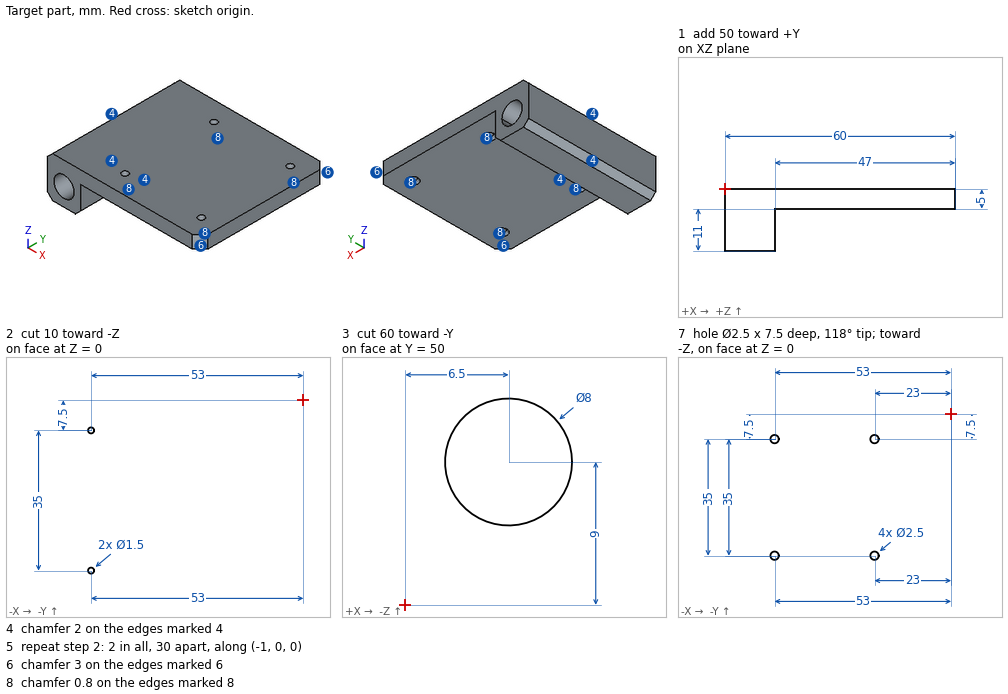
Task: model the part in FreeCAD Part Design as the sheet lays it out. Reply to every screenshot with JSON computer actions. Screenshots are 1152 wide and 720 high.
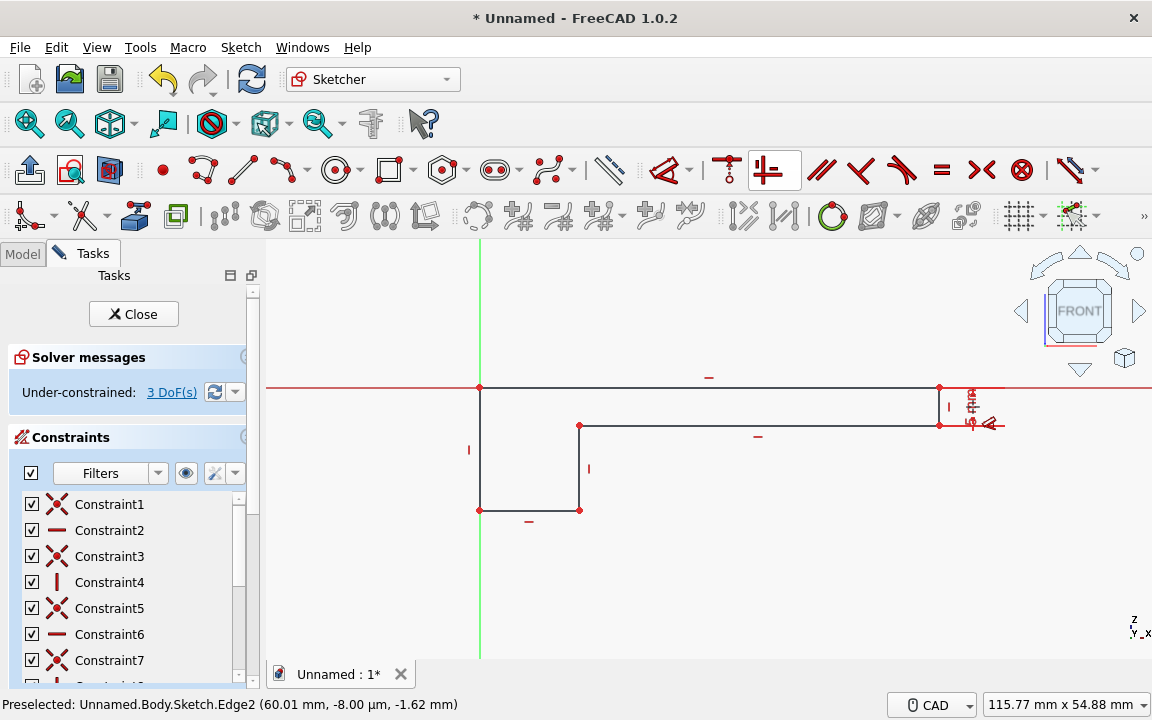
{"action": "left_click", "coordinate": [618, 388]}
{"action": "left_click", "coordinate": [709, 354]}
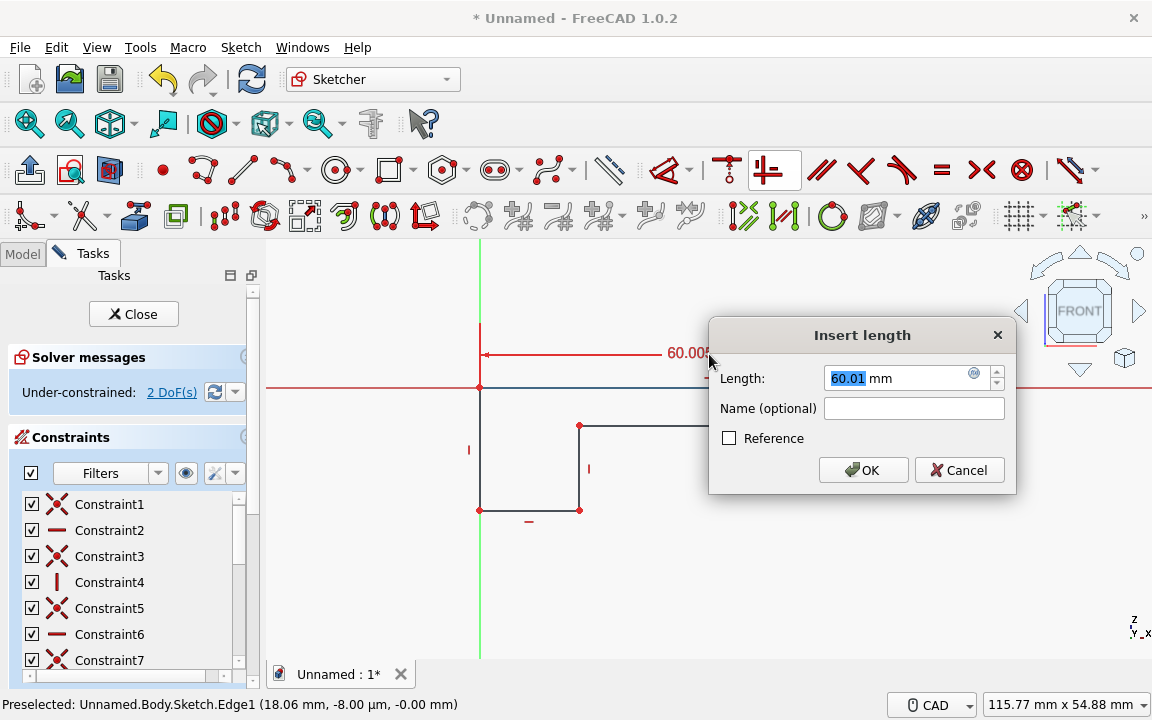
{"action": "type", "text": "60"}
{"action": "key", "text": "Return"}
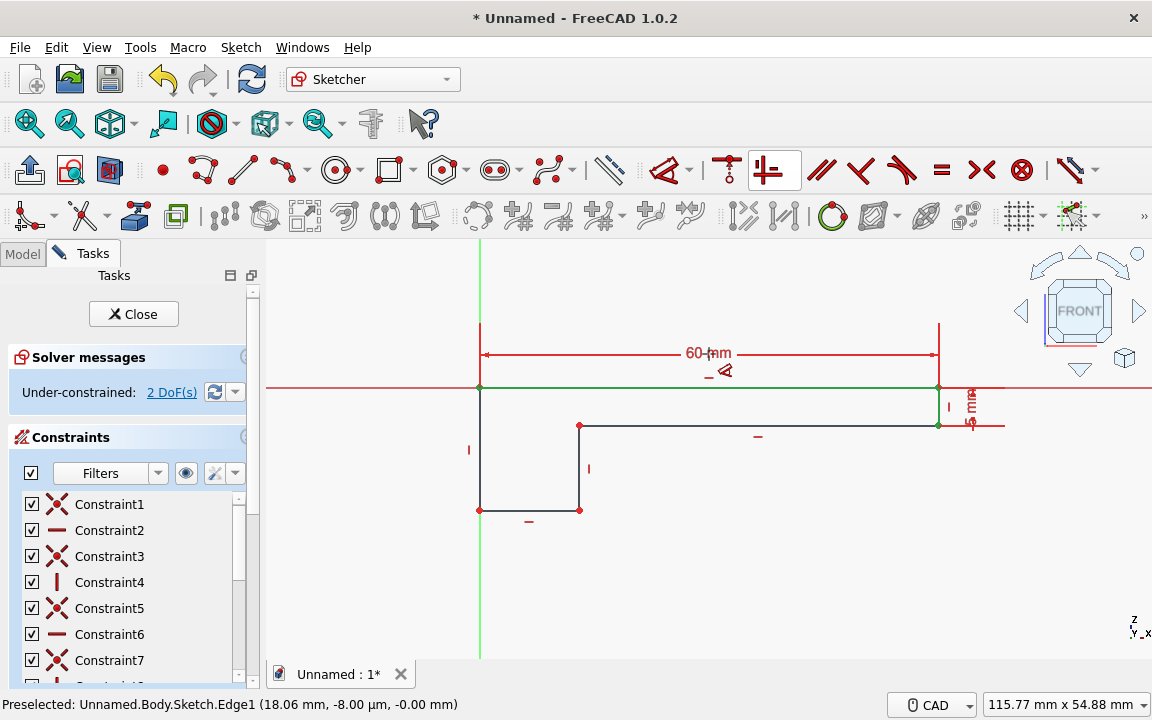
{"action": "left_click", "coordinate": [831, 426]}
{"action": "left_click", "coordinate": [759, 460]}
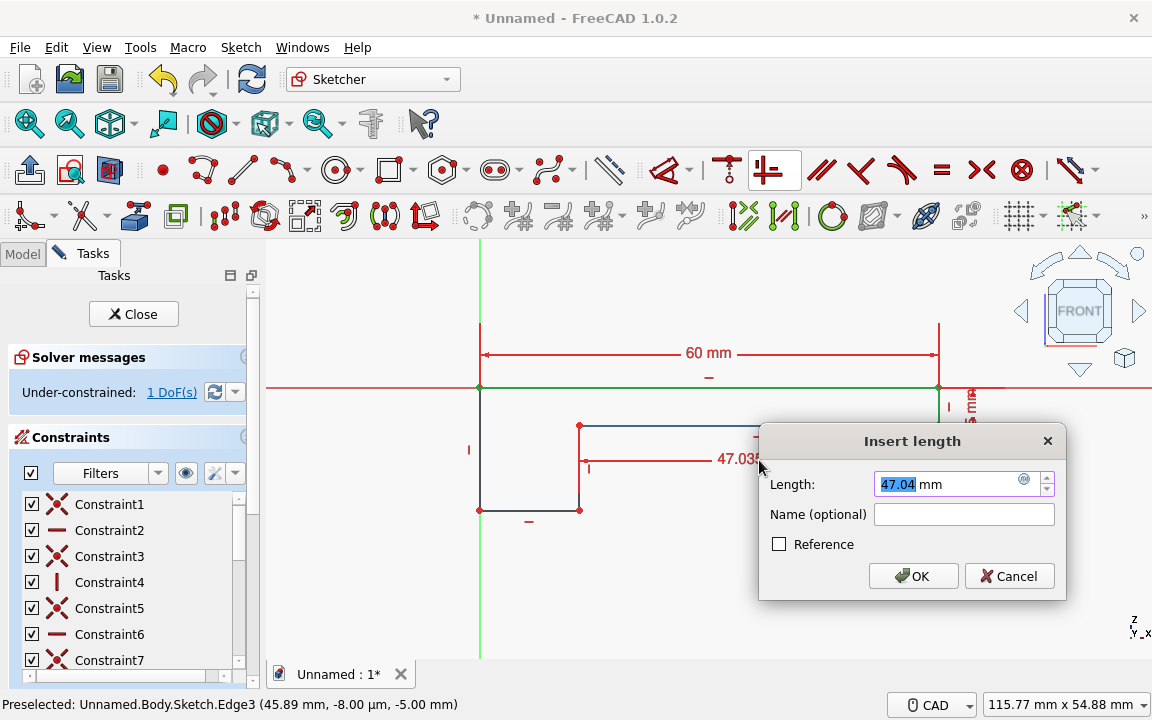
{"action": "type", "text": "47"}
{"action": "key", "text": "Return"}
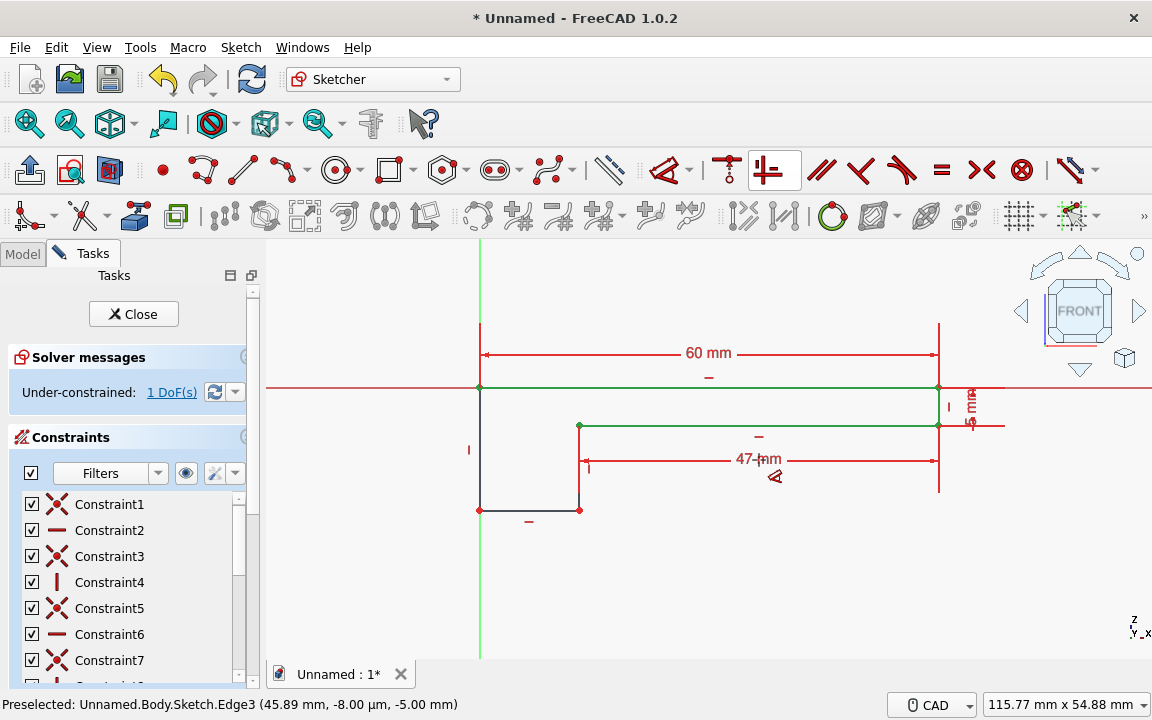
{"action": "left_click", "coordinate": [579, 451]}
{"action": "left_click", "coordinate": [545, 468]}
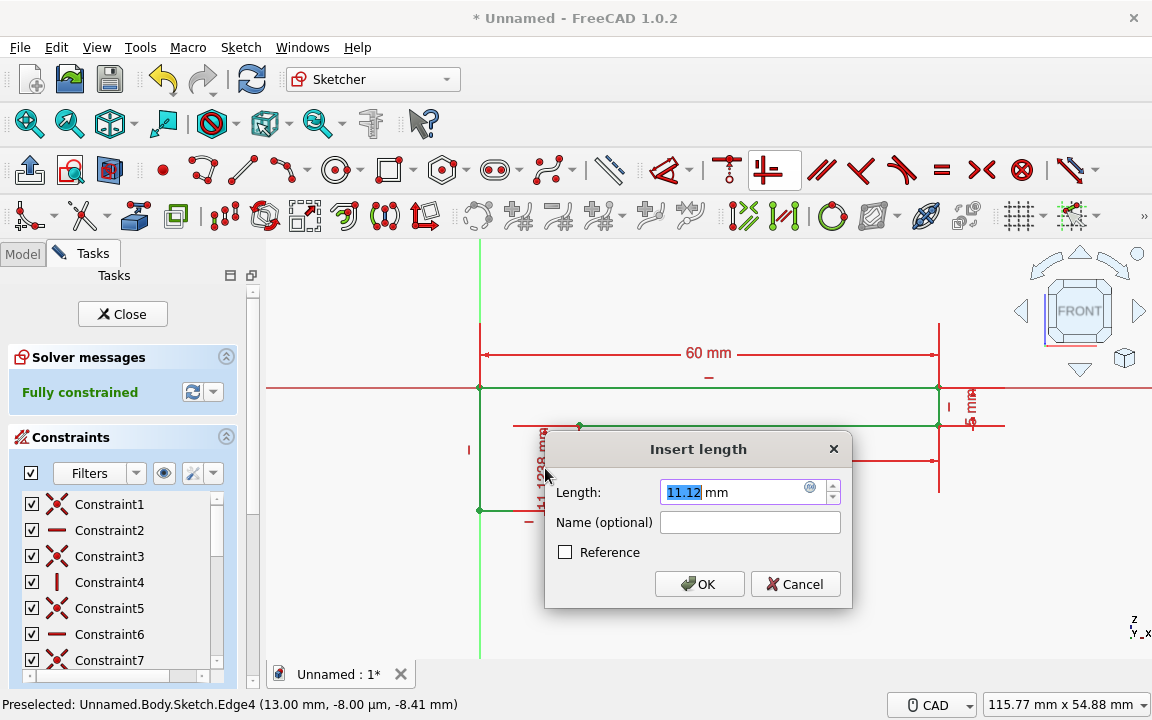
{"action": "type", "text": "11"}
{"action": "key", "text": "Return"}
{"action": "key", "text": "Escape"}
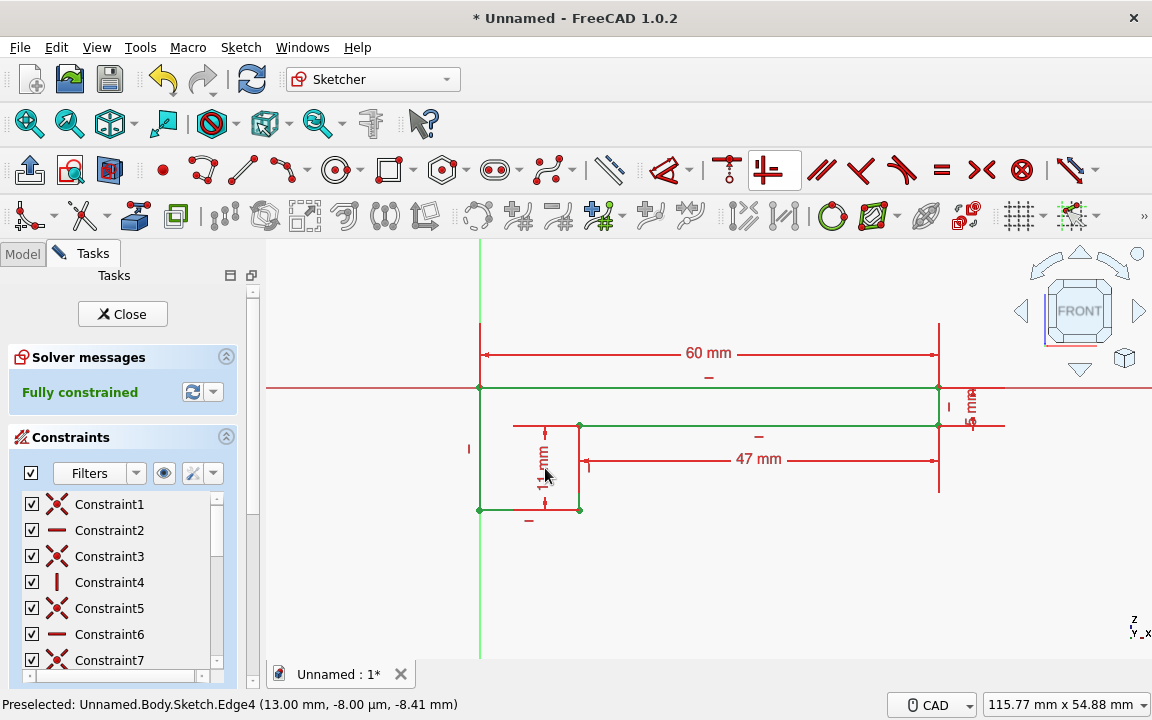
{"action": "left_click", "coordinate": [123, 314]}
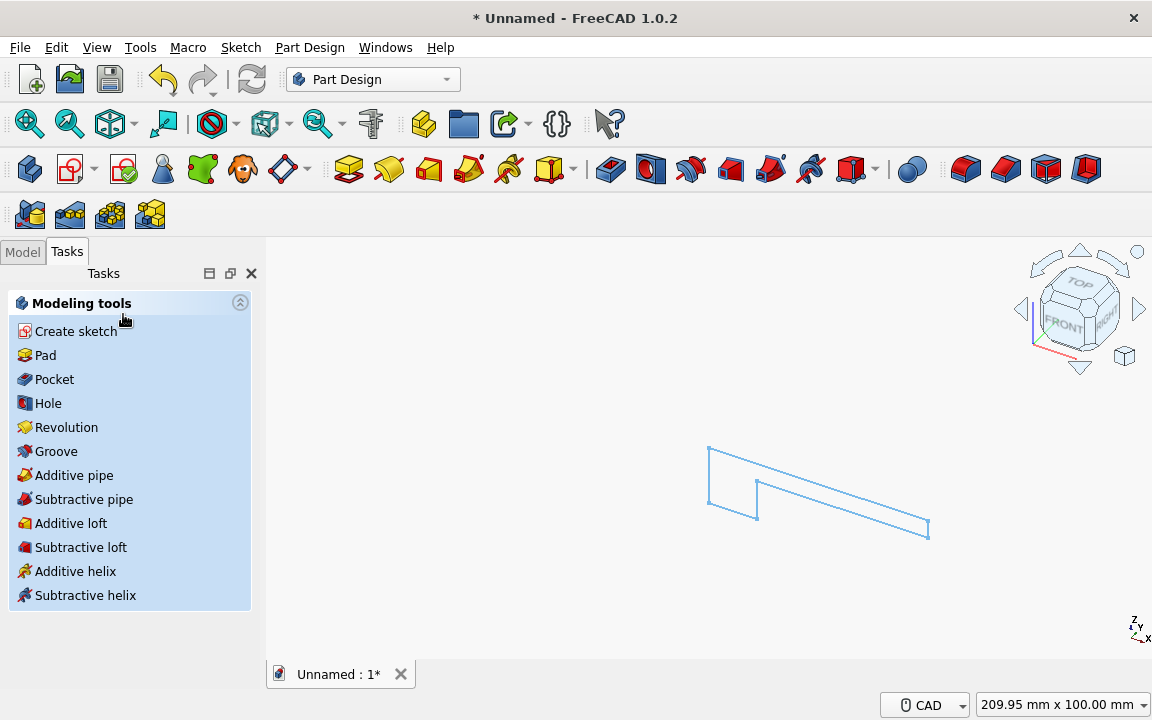
{"action": "left_click", "coordinate": [350, 170]}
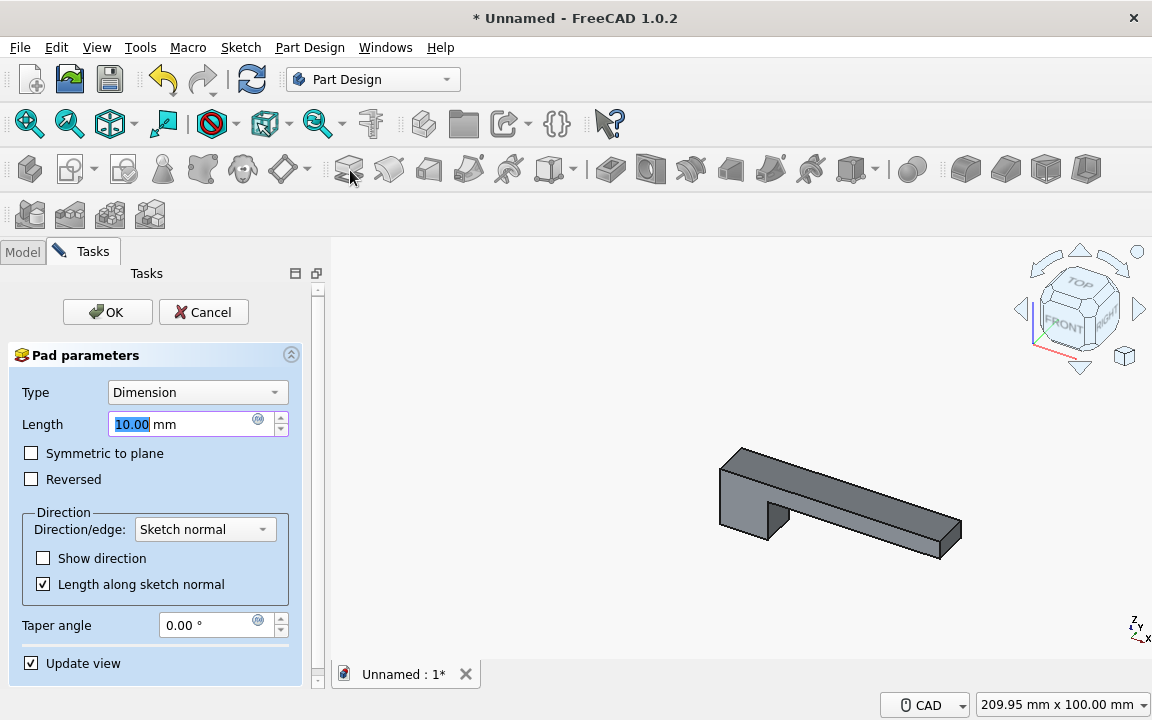
{"action": "type", "text": "50"}
{"action": "key", "text": "Tab"}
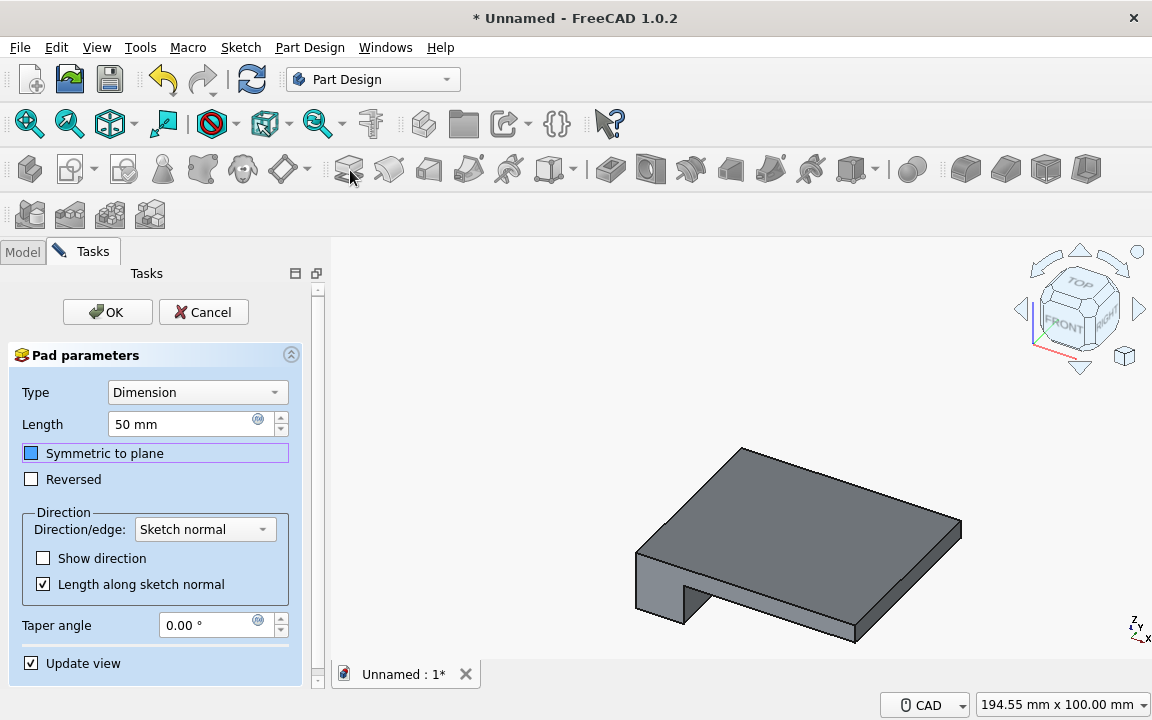
{"action": "left_click", "coordinate": [30, 479]}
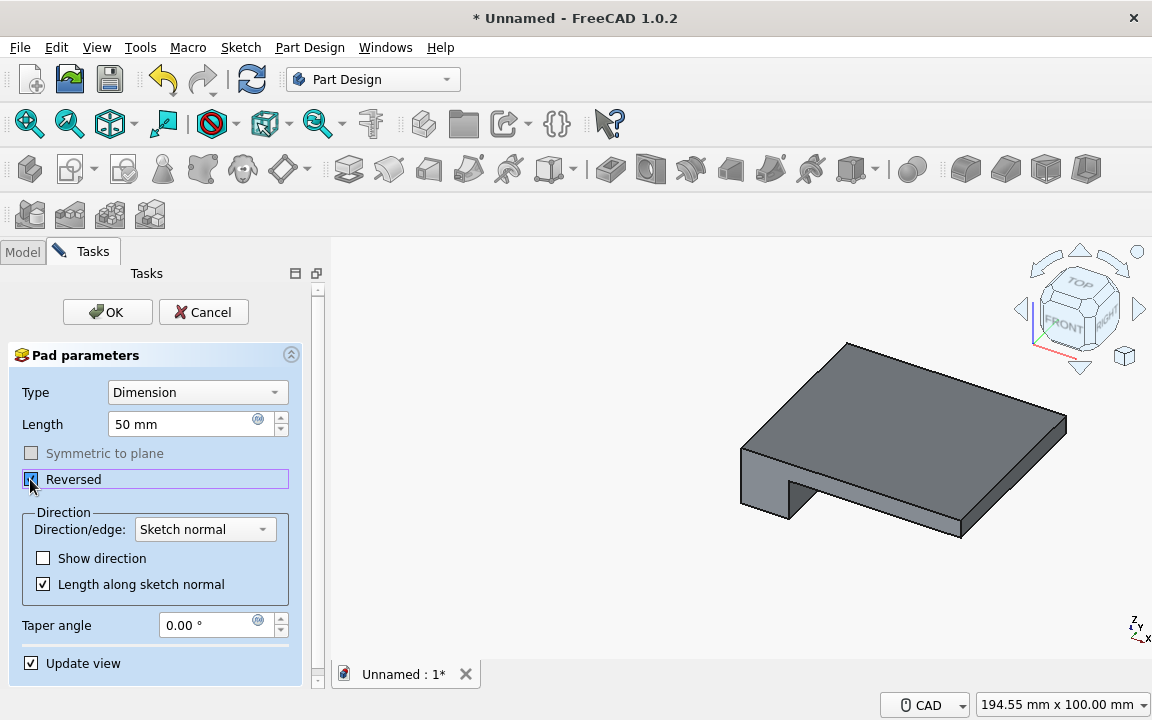
{"action": "left_click", "coordinate": [108, 312]}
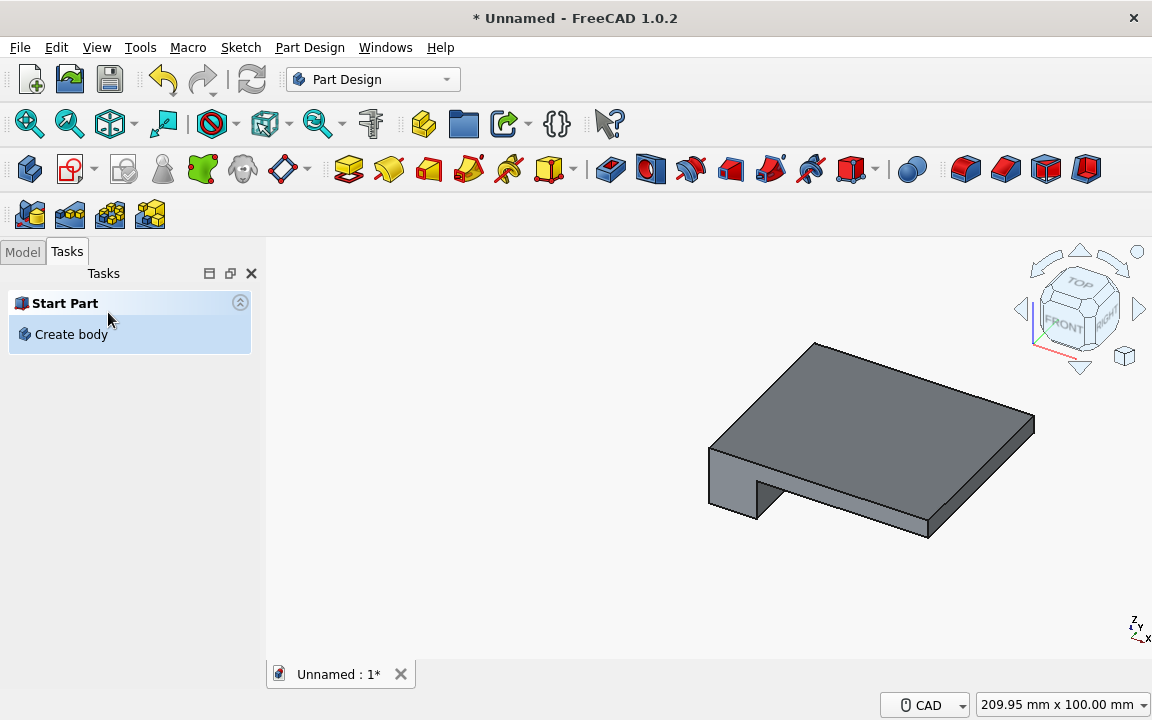
{"action": "left_click", "coordinate": [871, 431]}